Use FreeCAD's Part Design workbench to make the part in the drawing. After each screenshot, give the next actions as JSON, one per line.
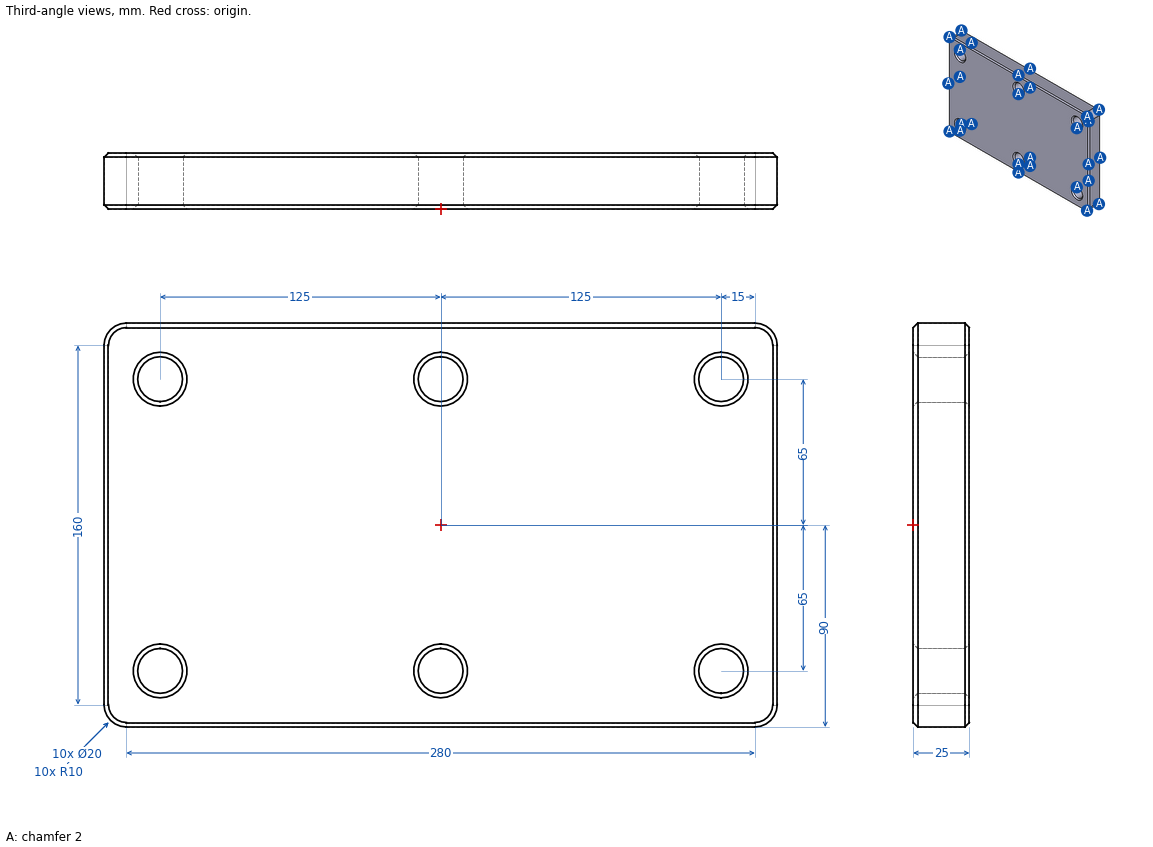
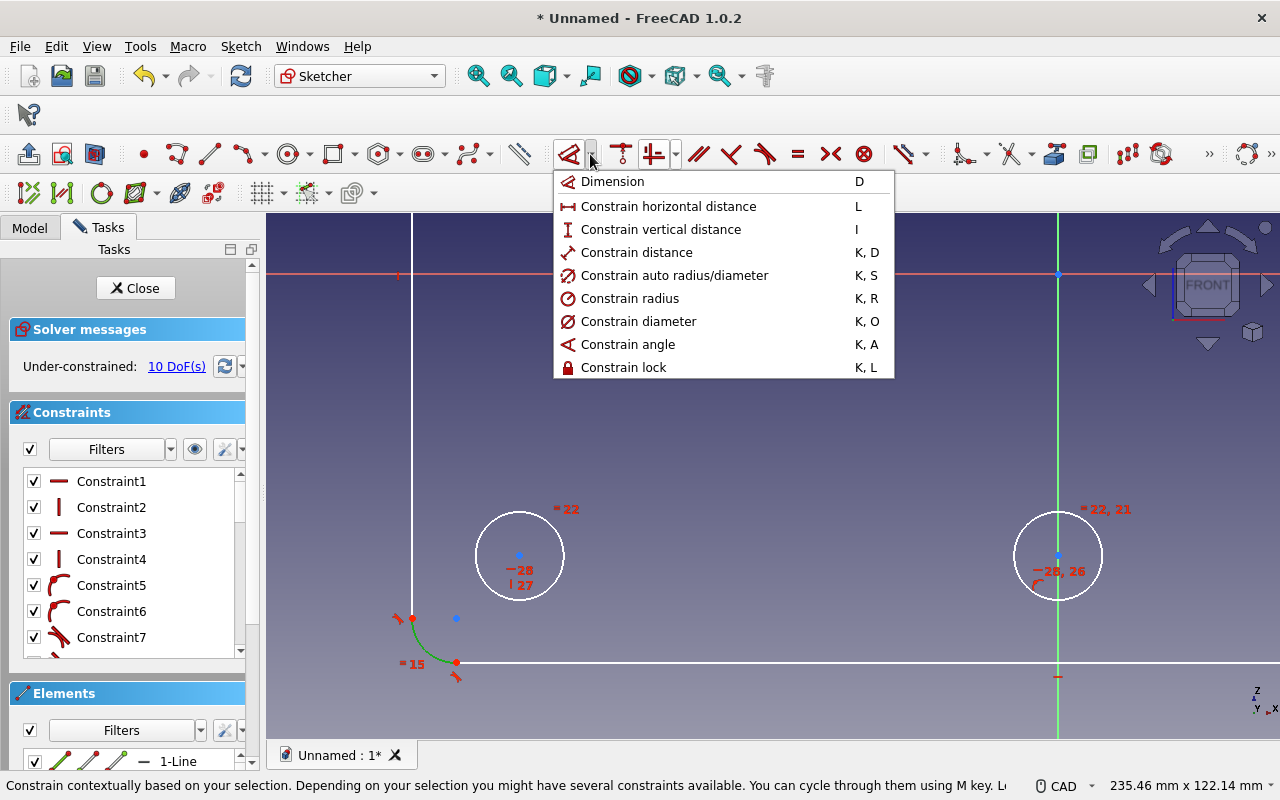
{"action": "left_click", "coordinate": [724, 298]}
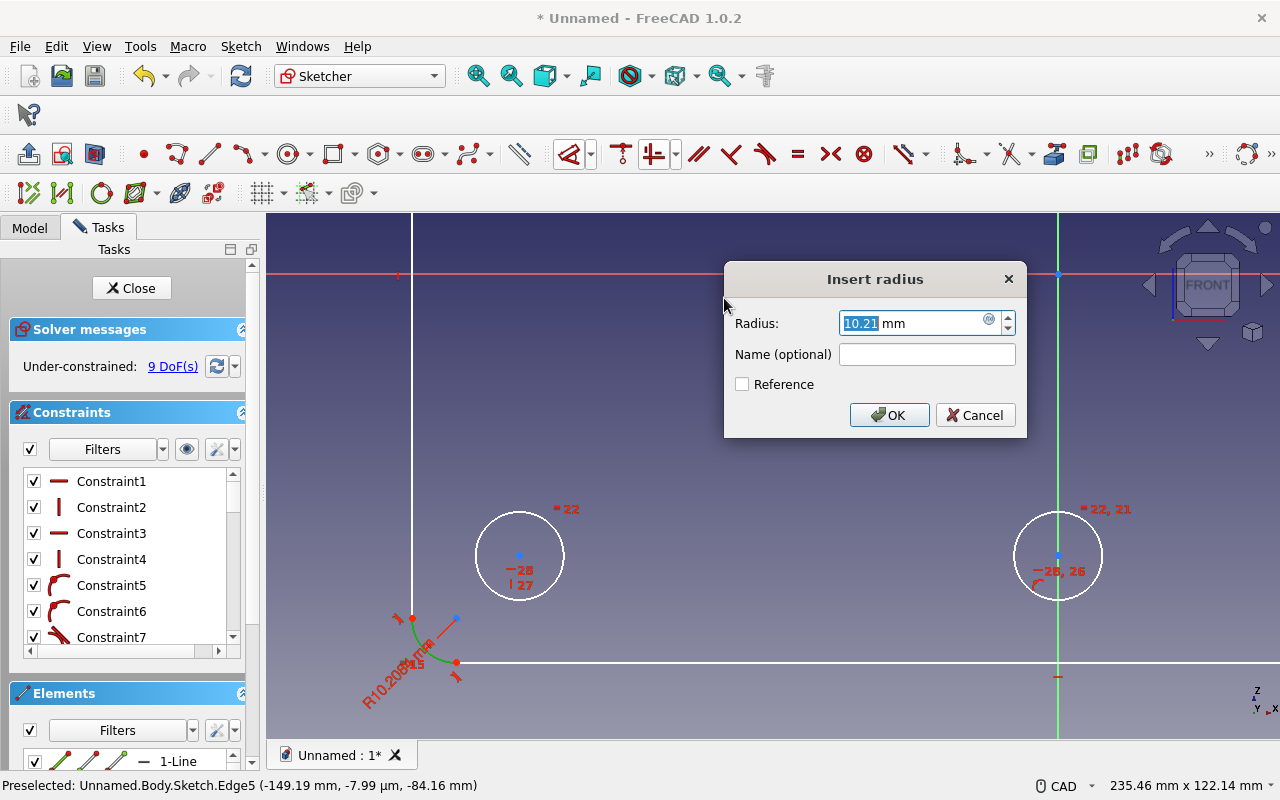
{"action": "type", "text": "10"}
{"action": "key", "text": "Return"}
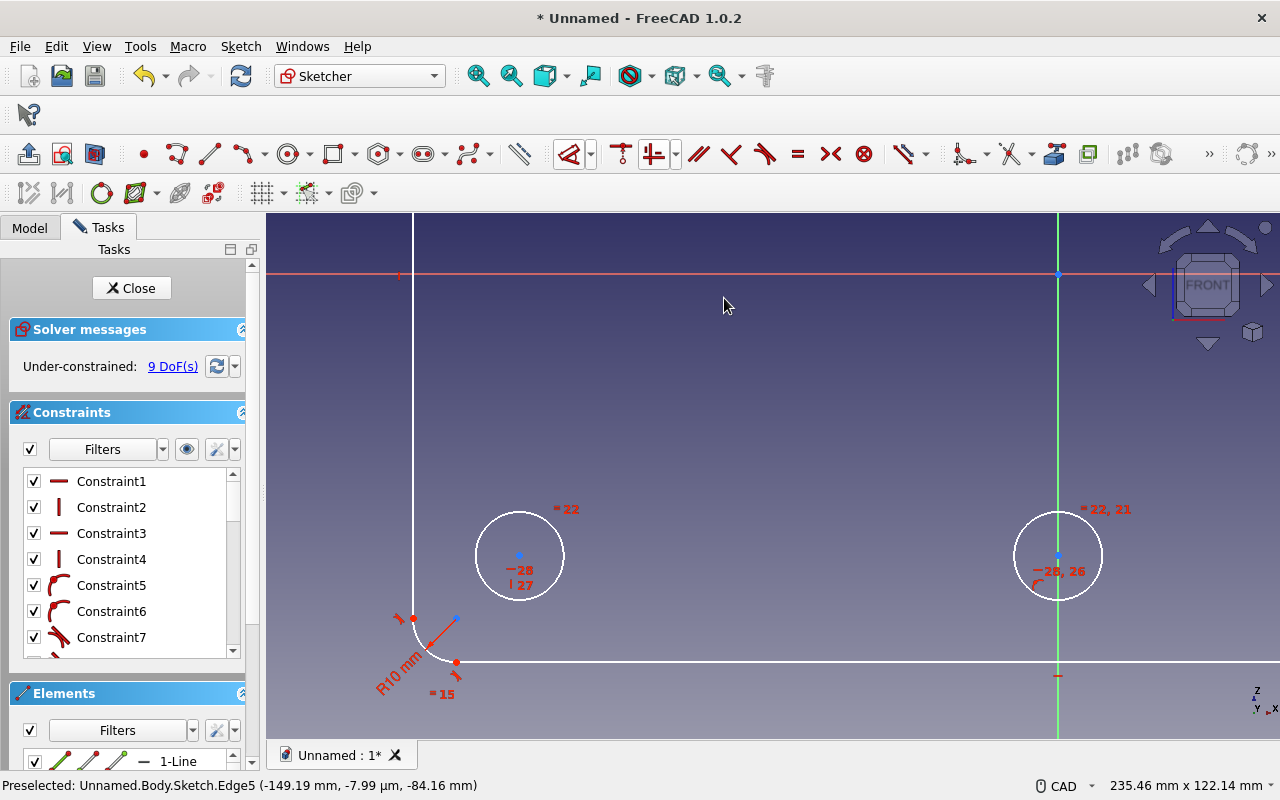
{"action": "scroll", "coordinate": [416, 641], "scroll_direction": "down", "scroll_amount": 4}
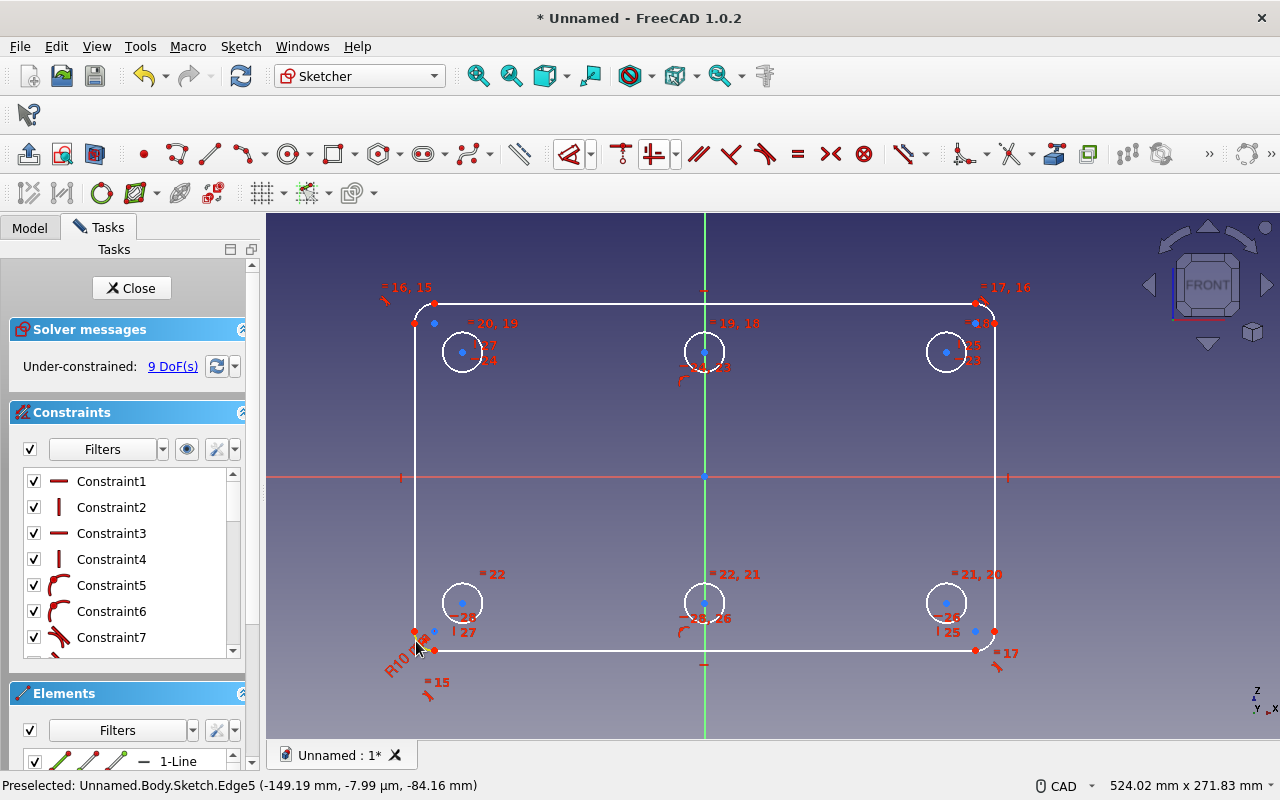
{"action": "left_click", "coordinate": [933, 338]}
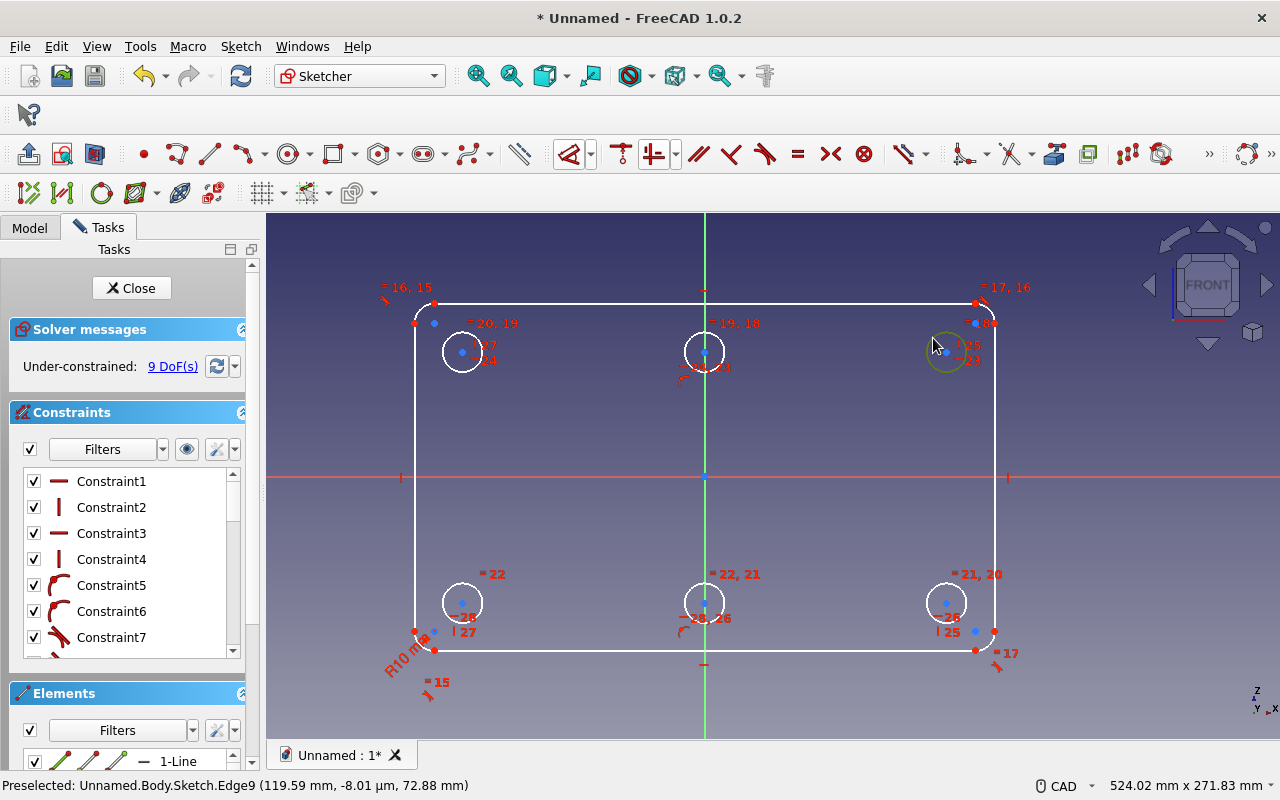
{"action": "left_click", "coordinate": [590, 154]}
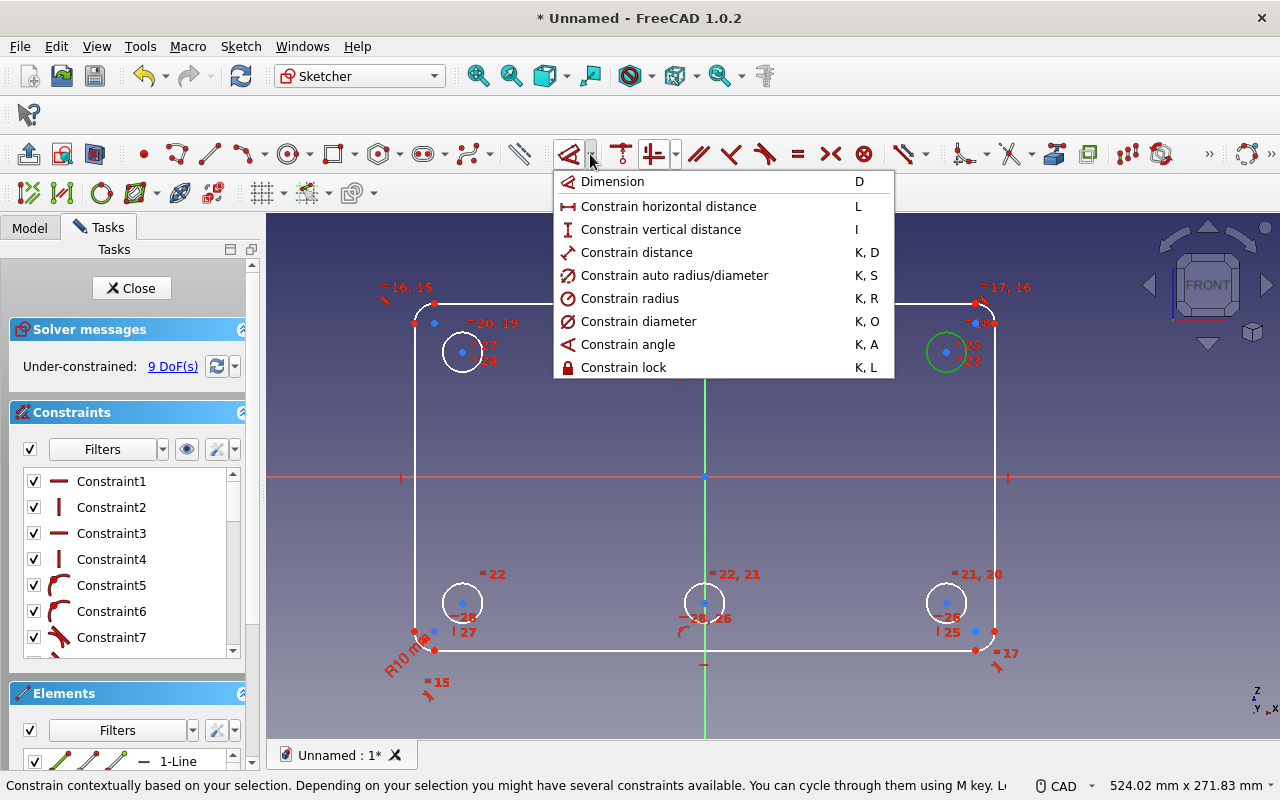
{"action": "left_click", "coordinate": [724, 322]}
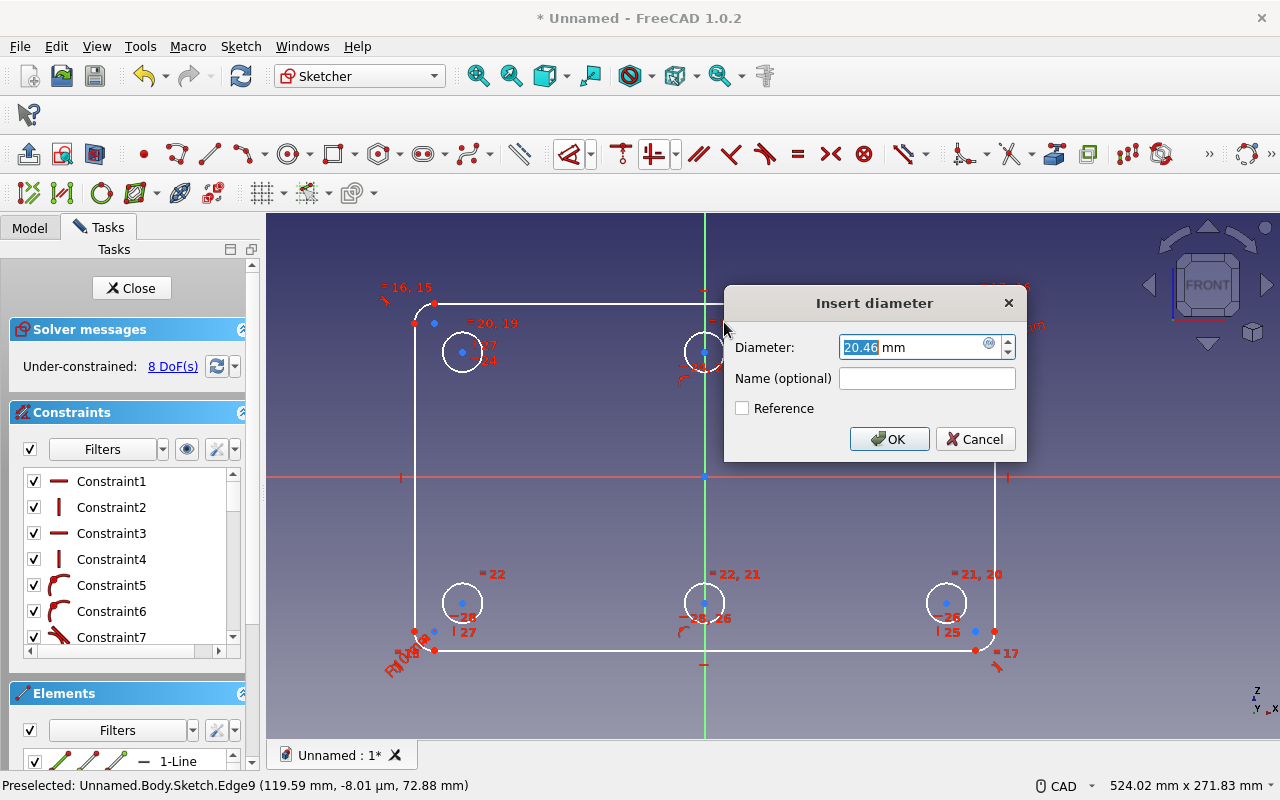
{"action": "type", "text": "20"}
{"action": "key", "text": "Return"}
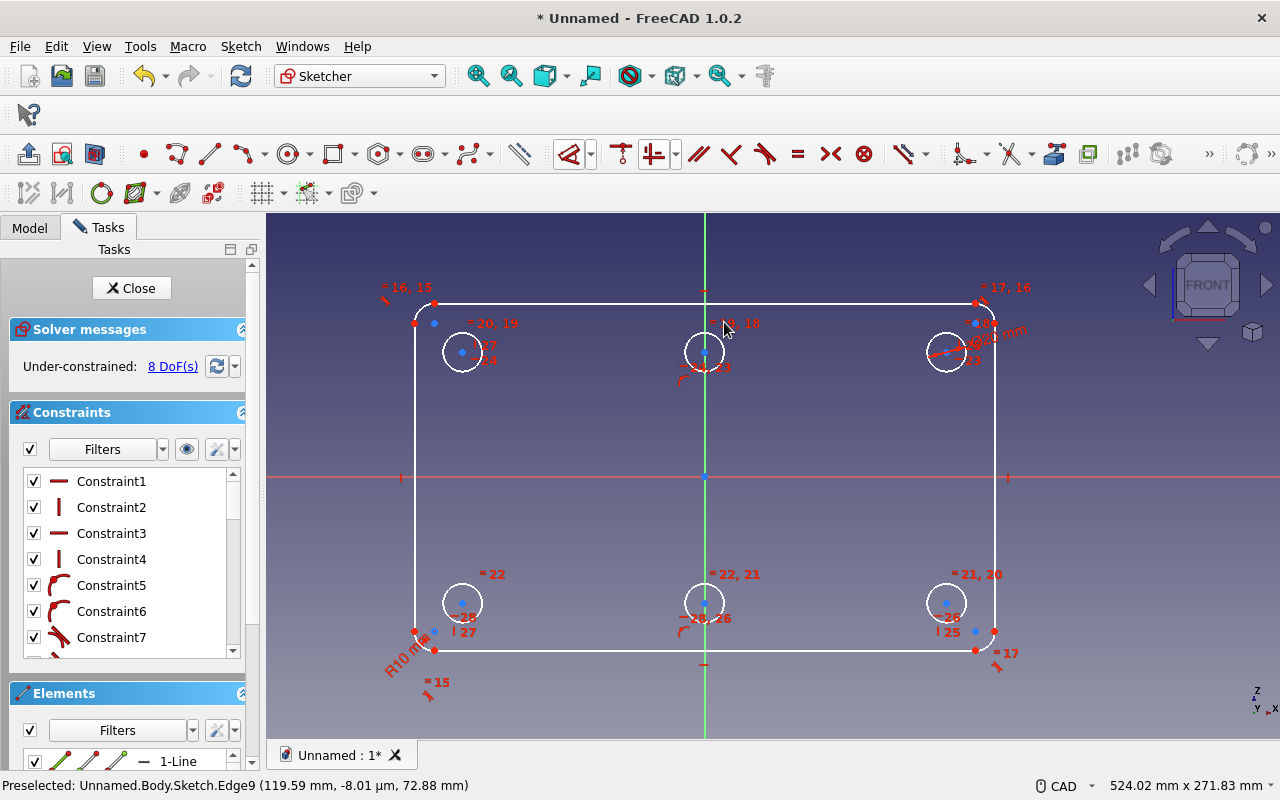
{"action": "left_click", "coordinate": [947, 352]}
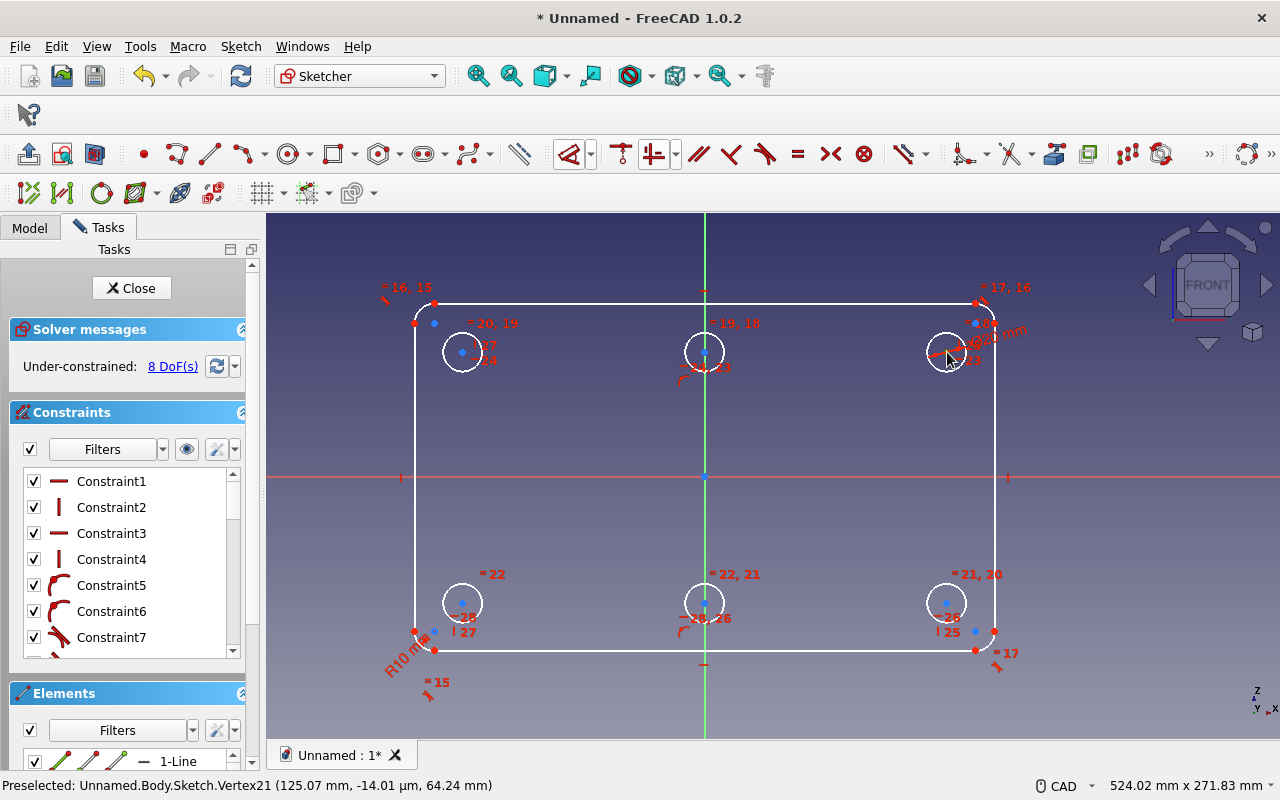
{"action": "key", "text": "i"}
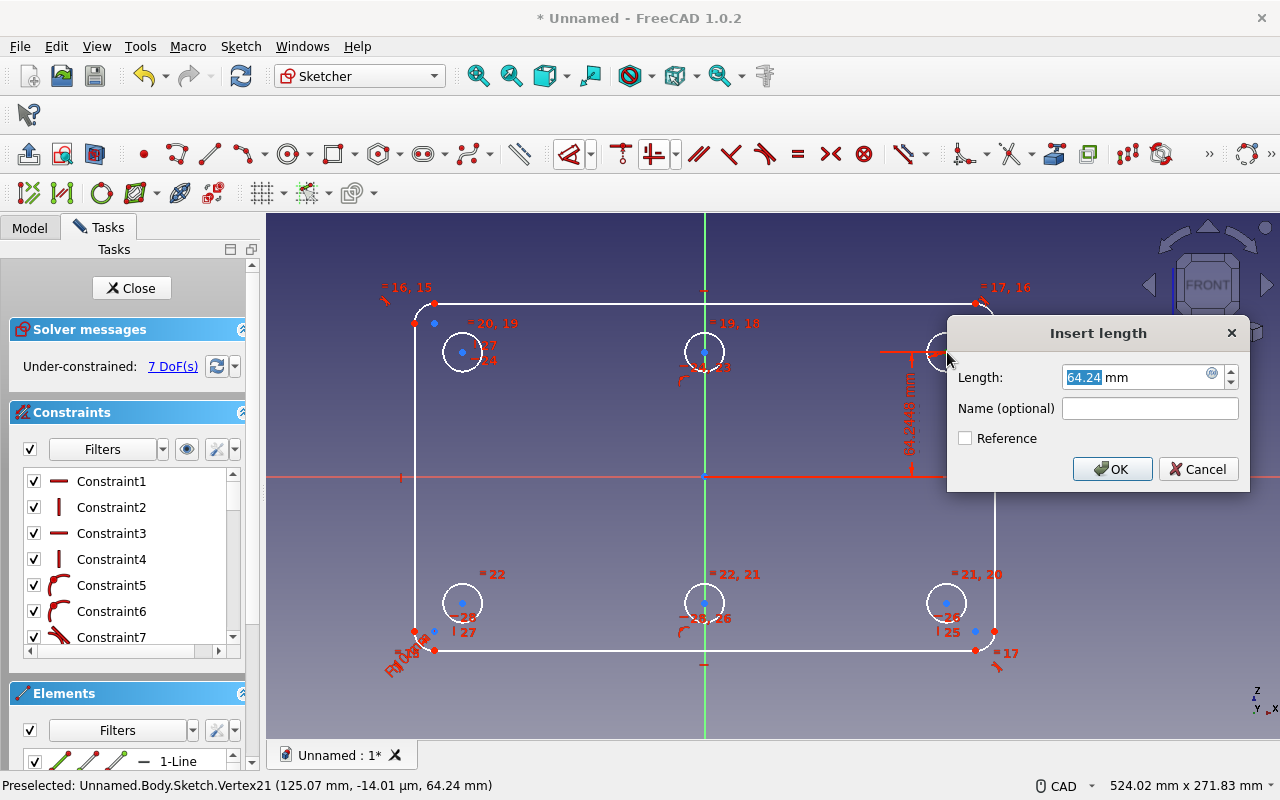
{"action": "type", "text": "65"}
{"action": "key", "text": "Return"}